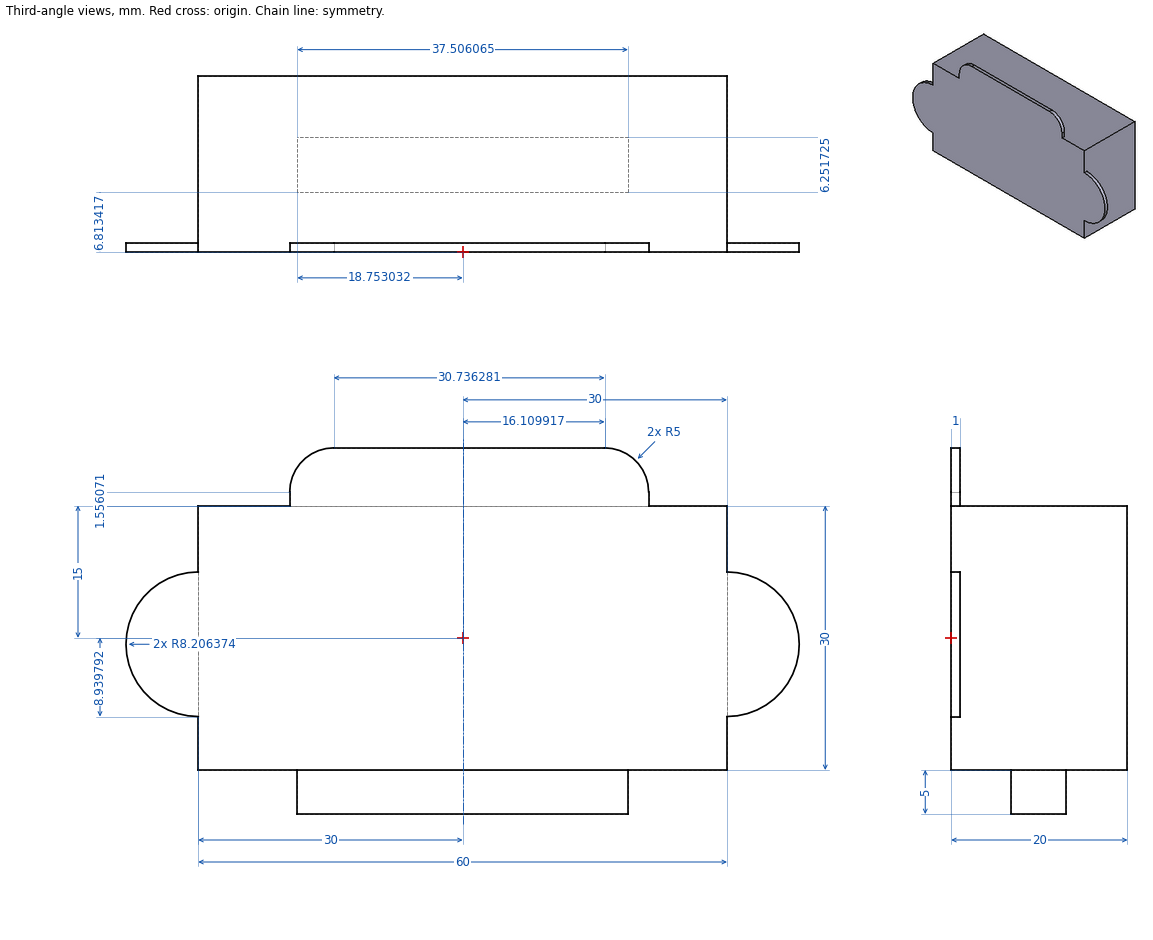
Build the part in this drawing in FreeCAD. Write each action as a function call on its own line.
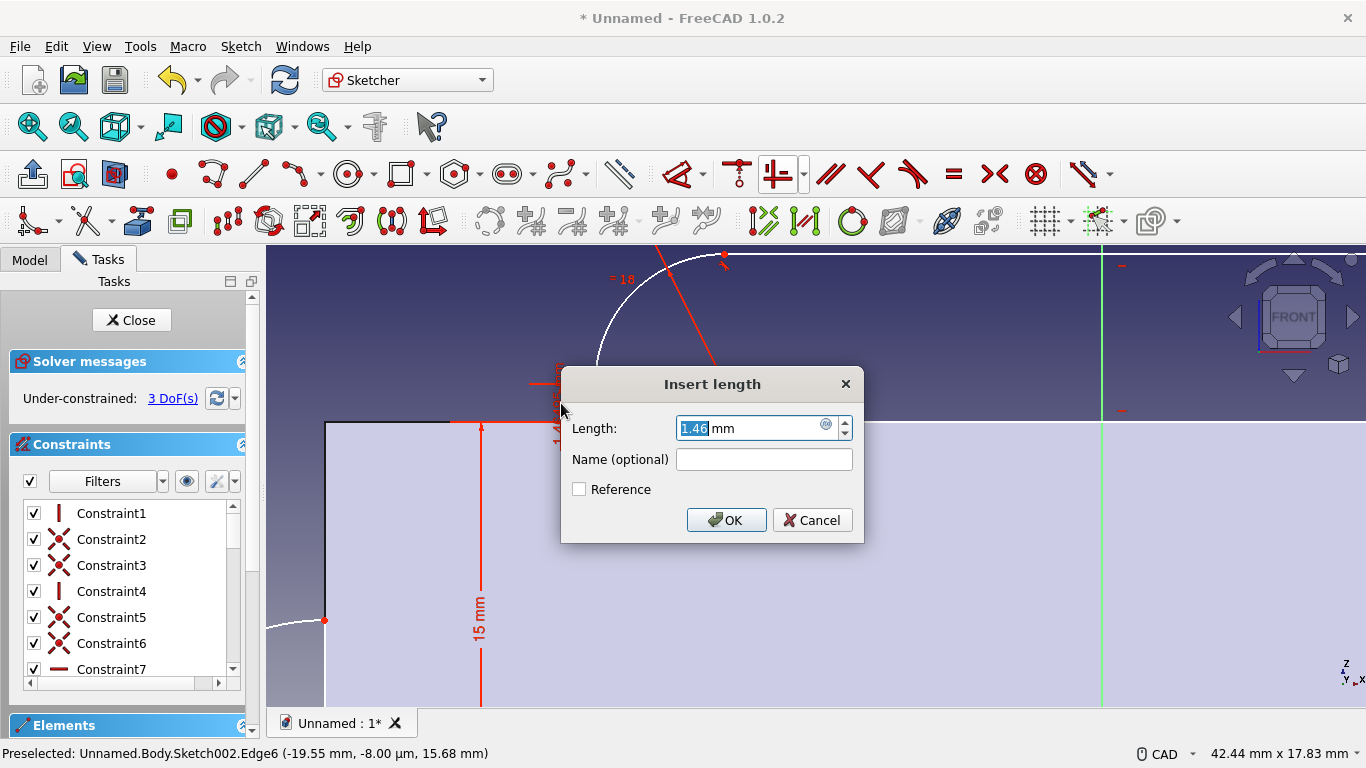
text(1.556071)
key(Return)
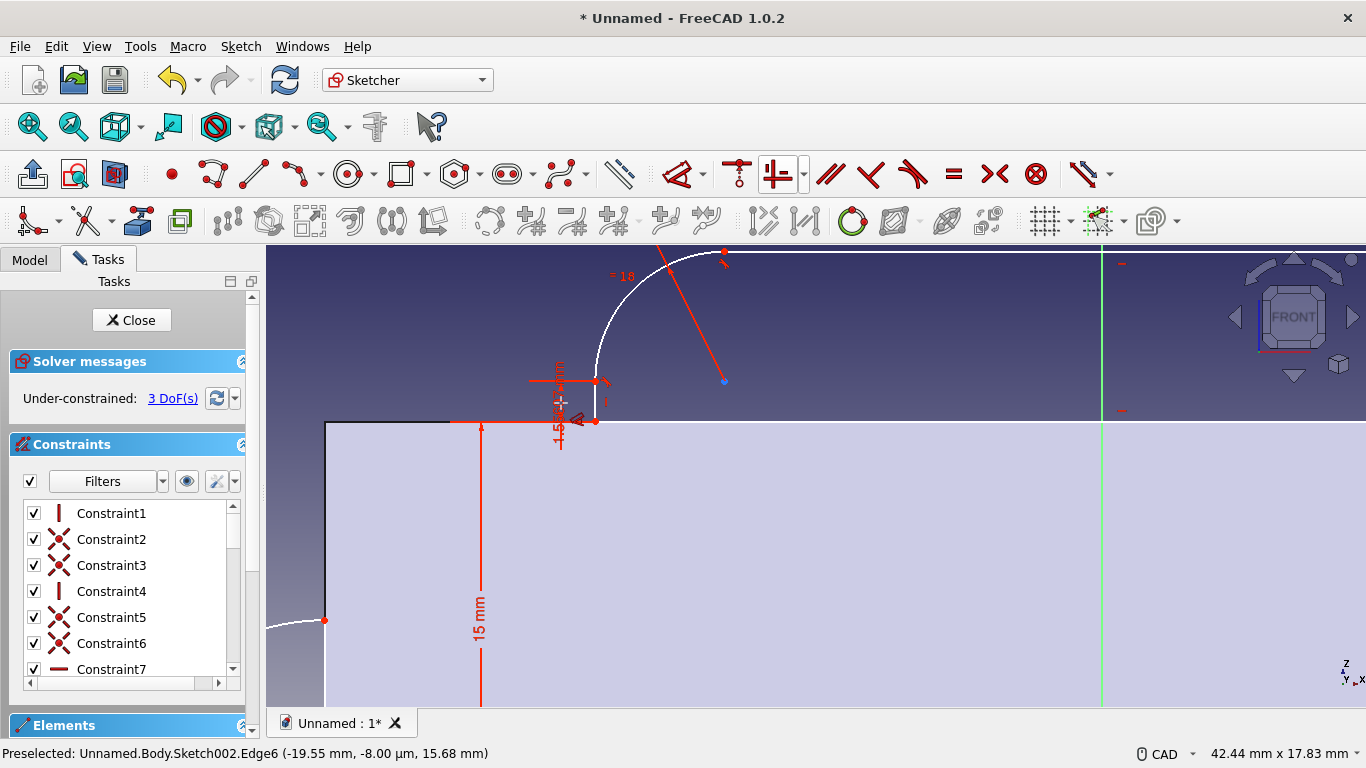
scroll(595, 402, down, 6)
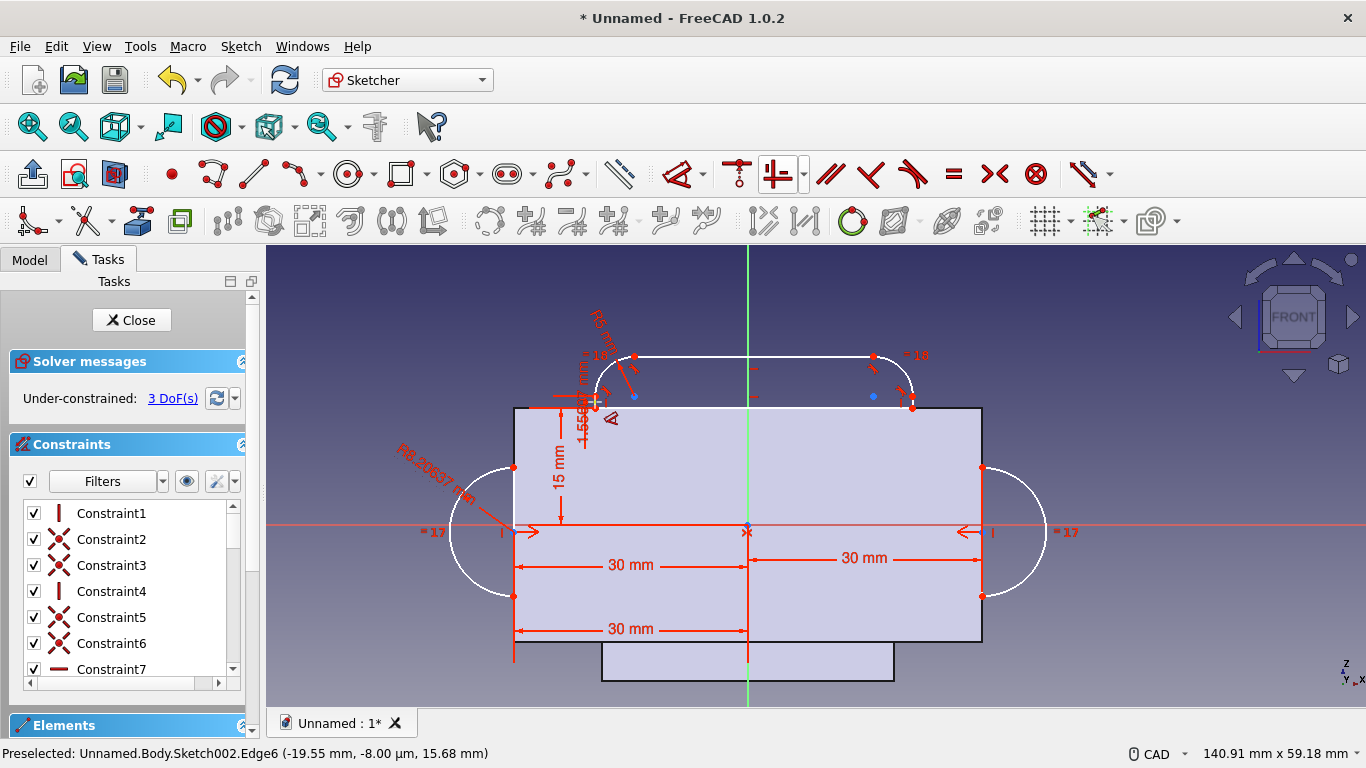
click(802, 357)
click(699, 323)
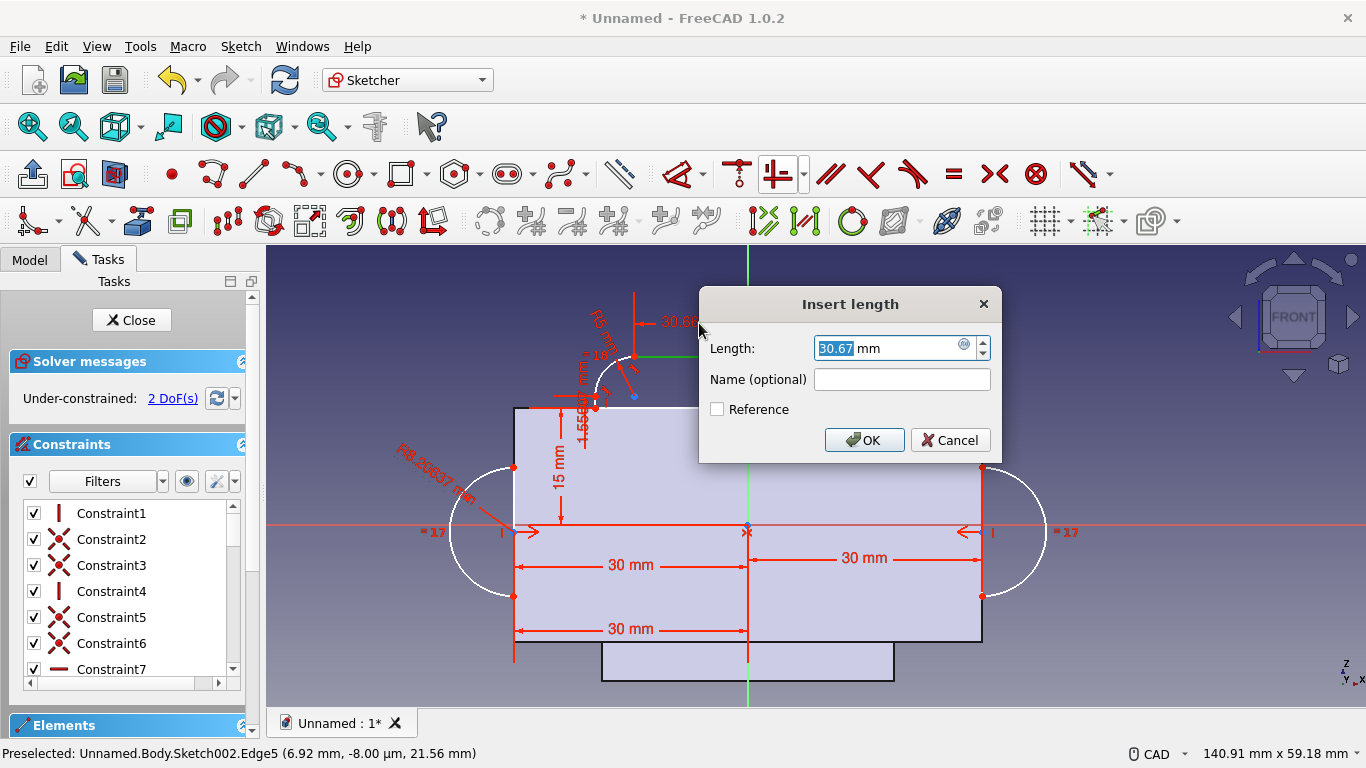
text(30.736281)
key(Return)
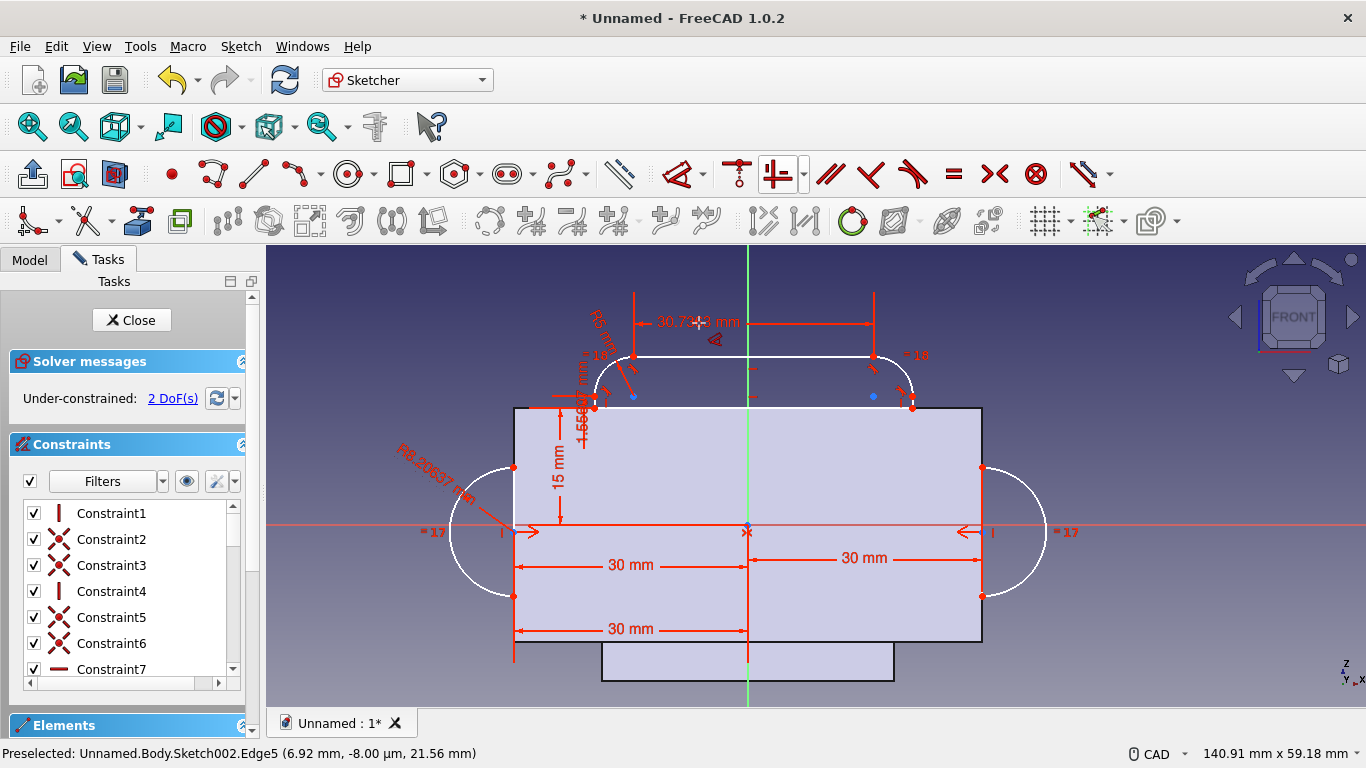
click(514, 596)
click(480, 561)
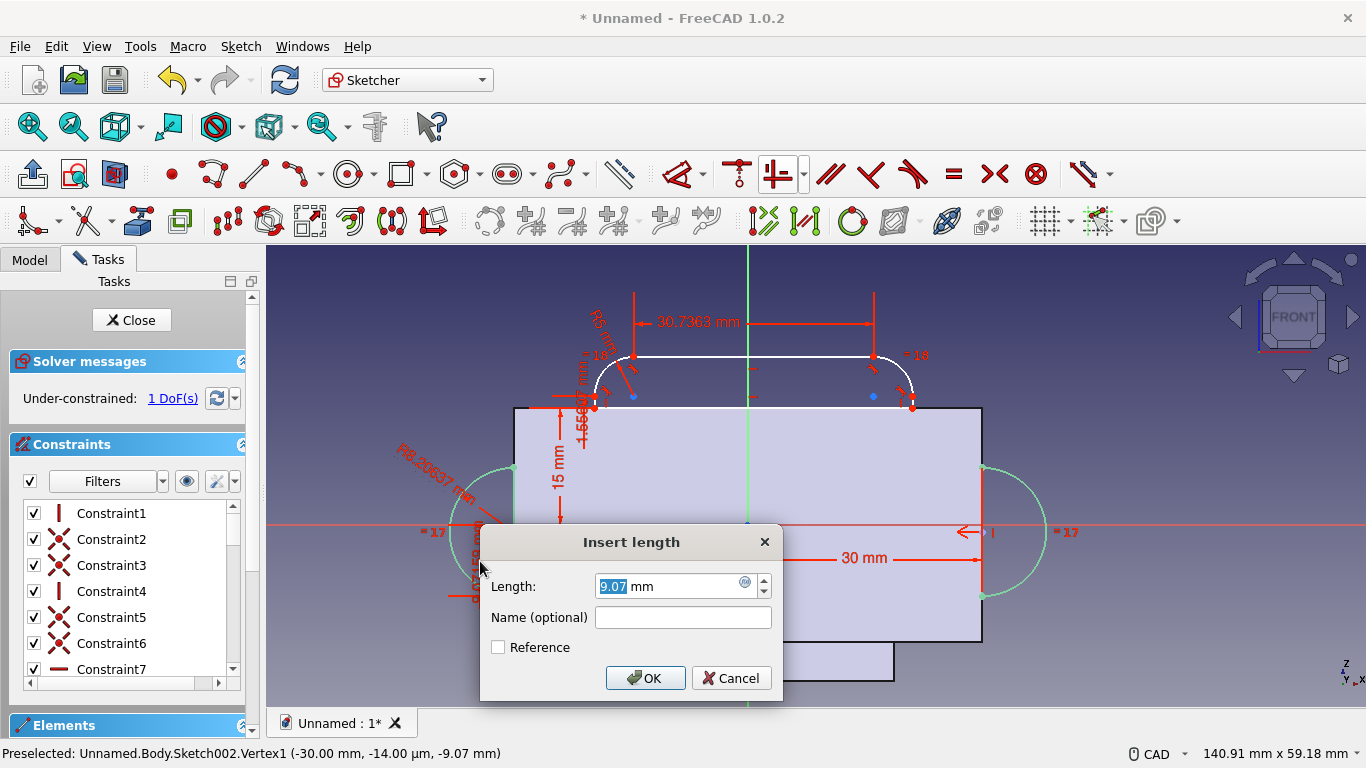
text(8.939792)
key(Return)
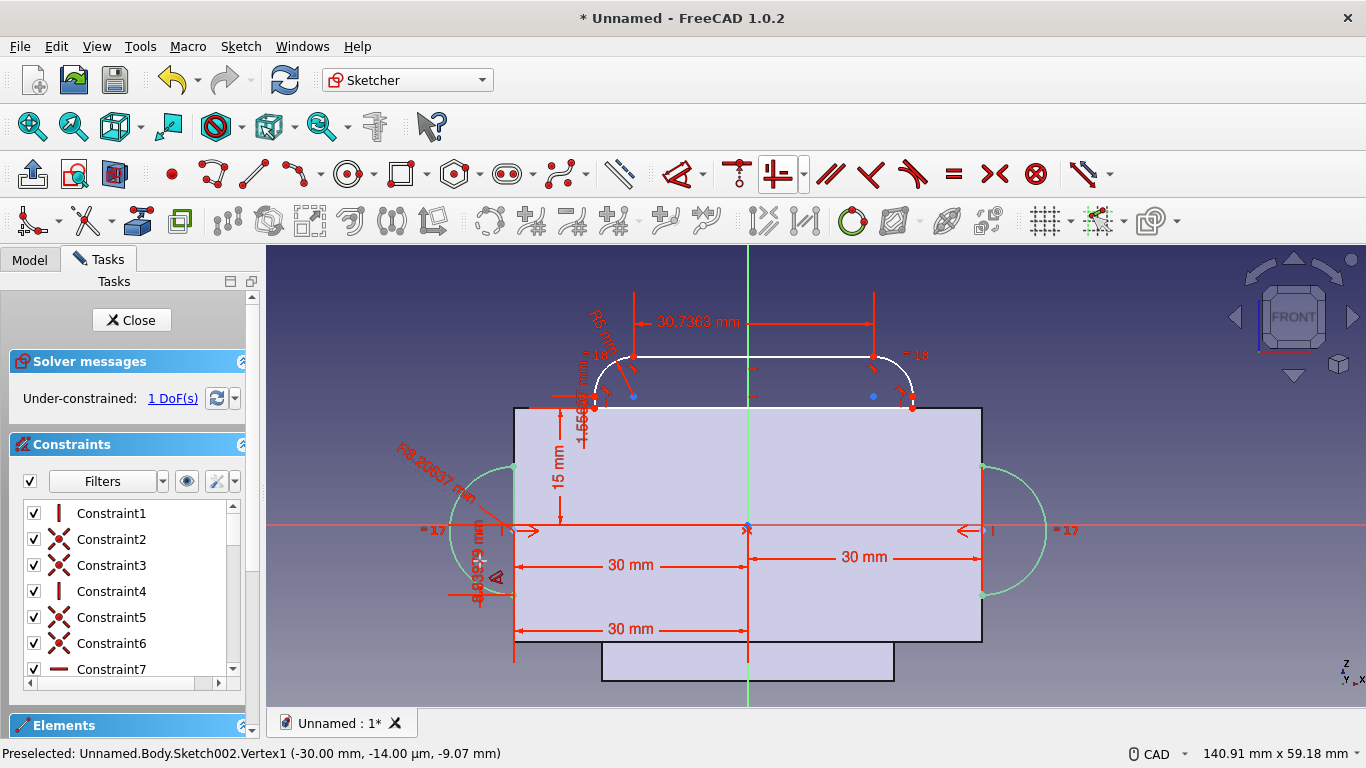
click(874, 357)
click(811, 323)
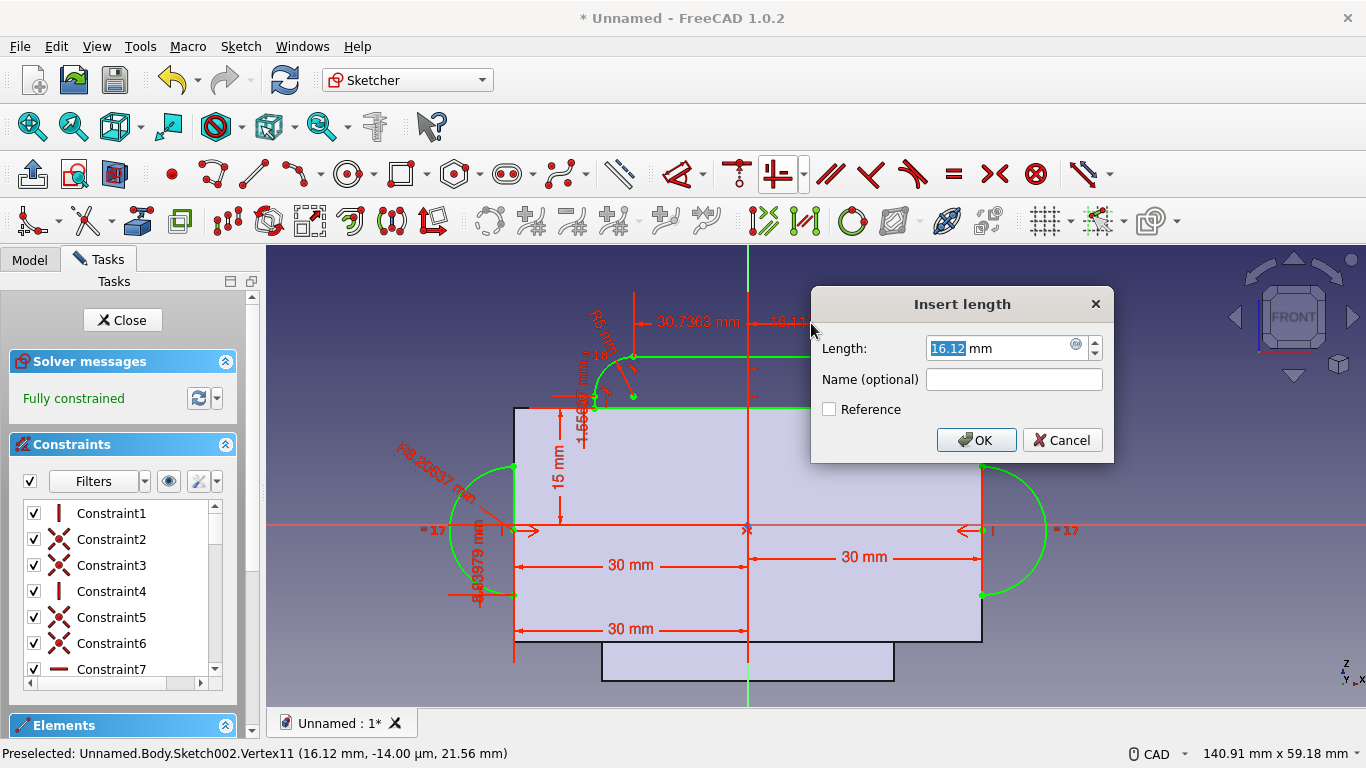
text(16.109917)
key(Return)
key(Escape)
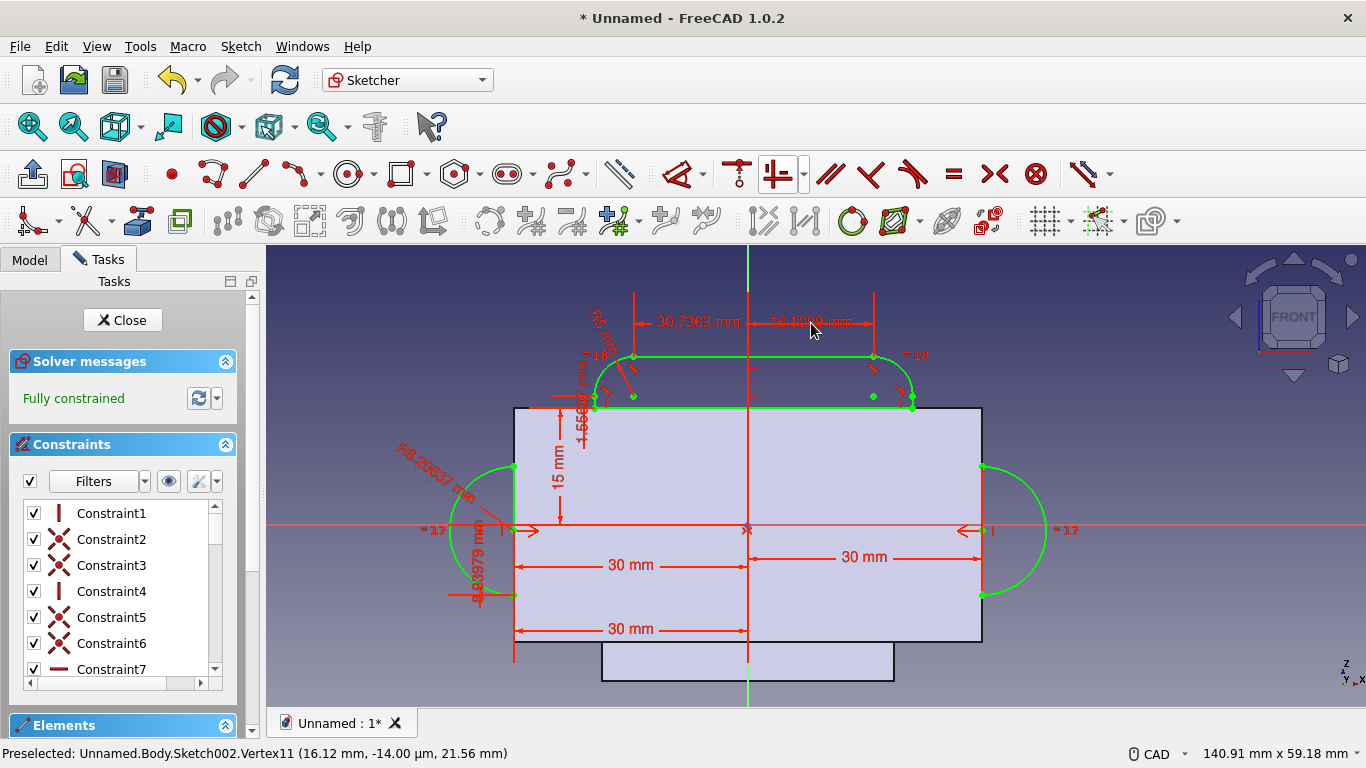
click(123, 320)